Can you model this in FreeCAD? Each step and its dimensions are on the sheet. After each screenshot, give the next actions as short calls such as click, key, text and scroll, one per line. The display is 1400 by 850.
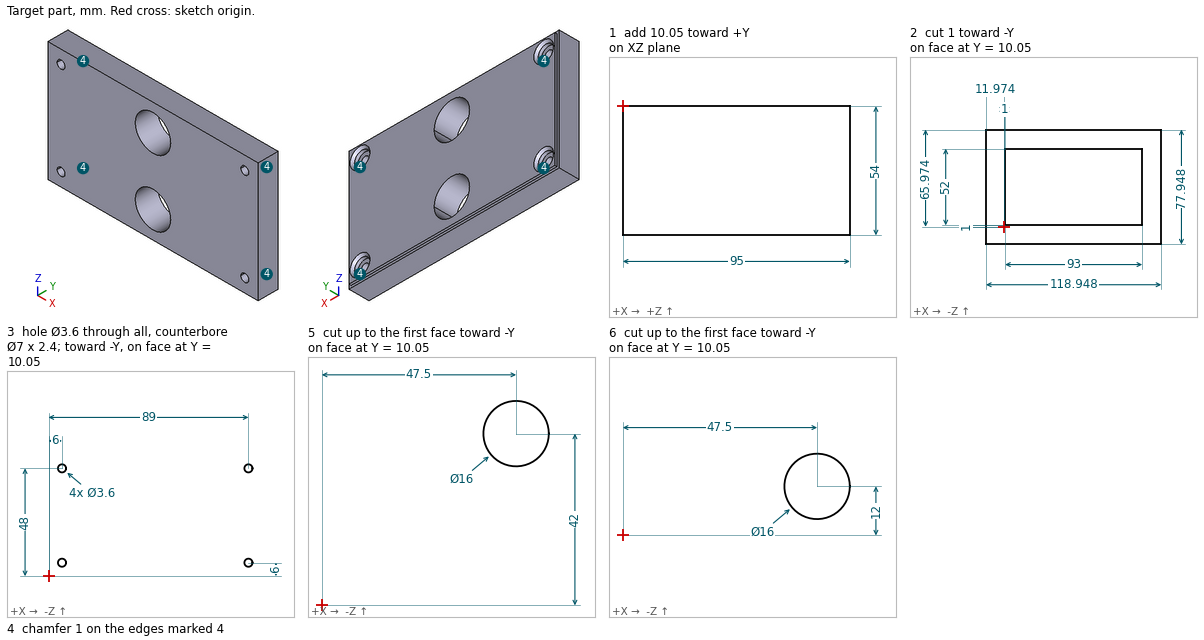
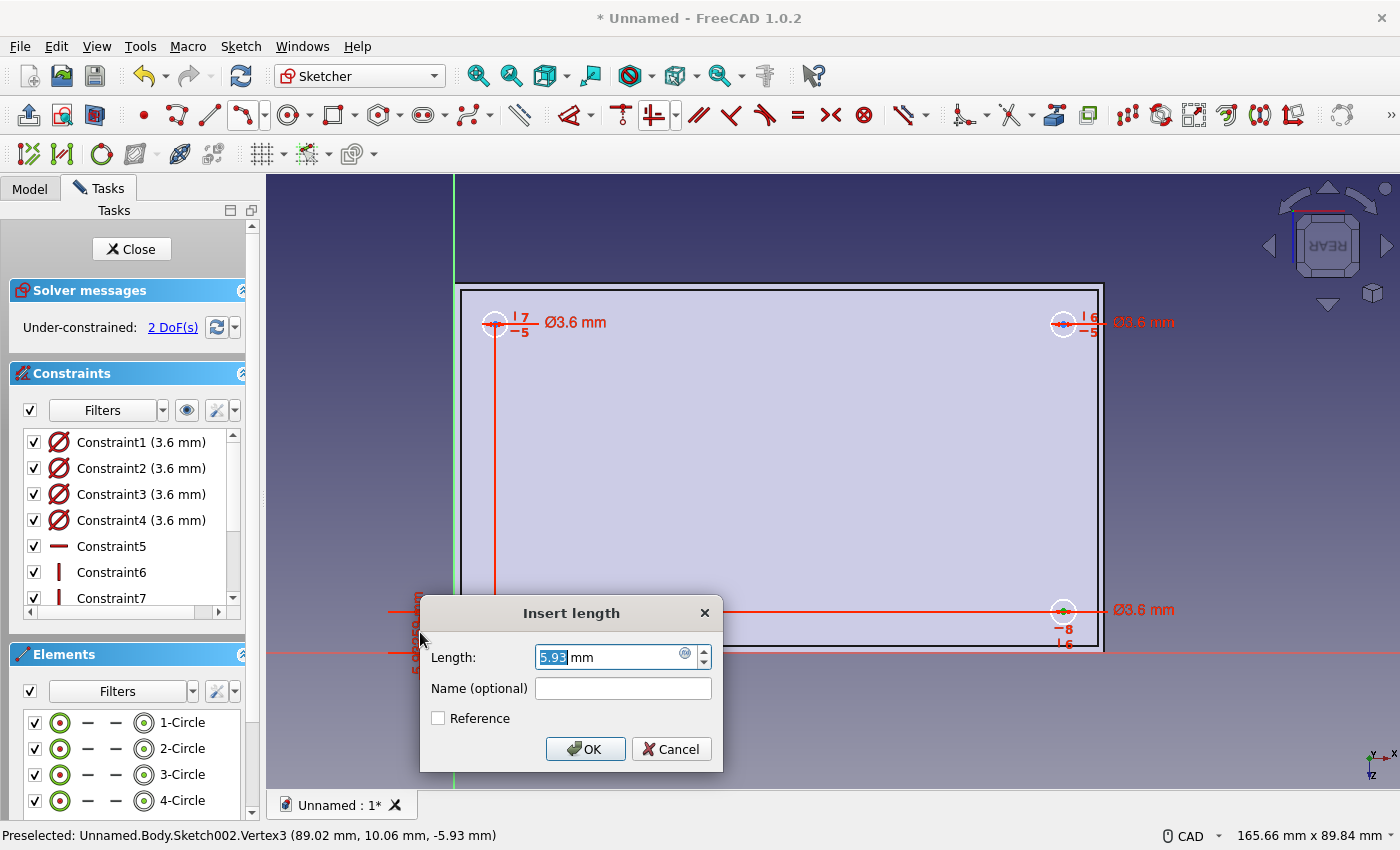
text(6)
key(Return)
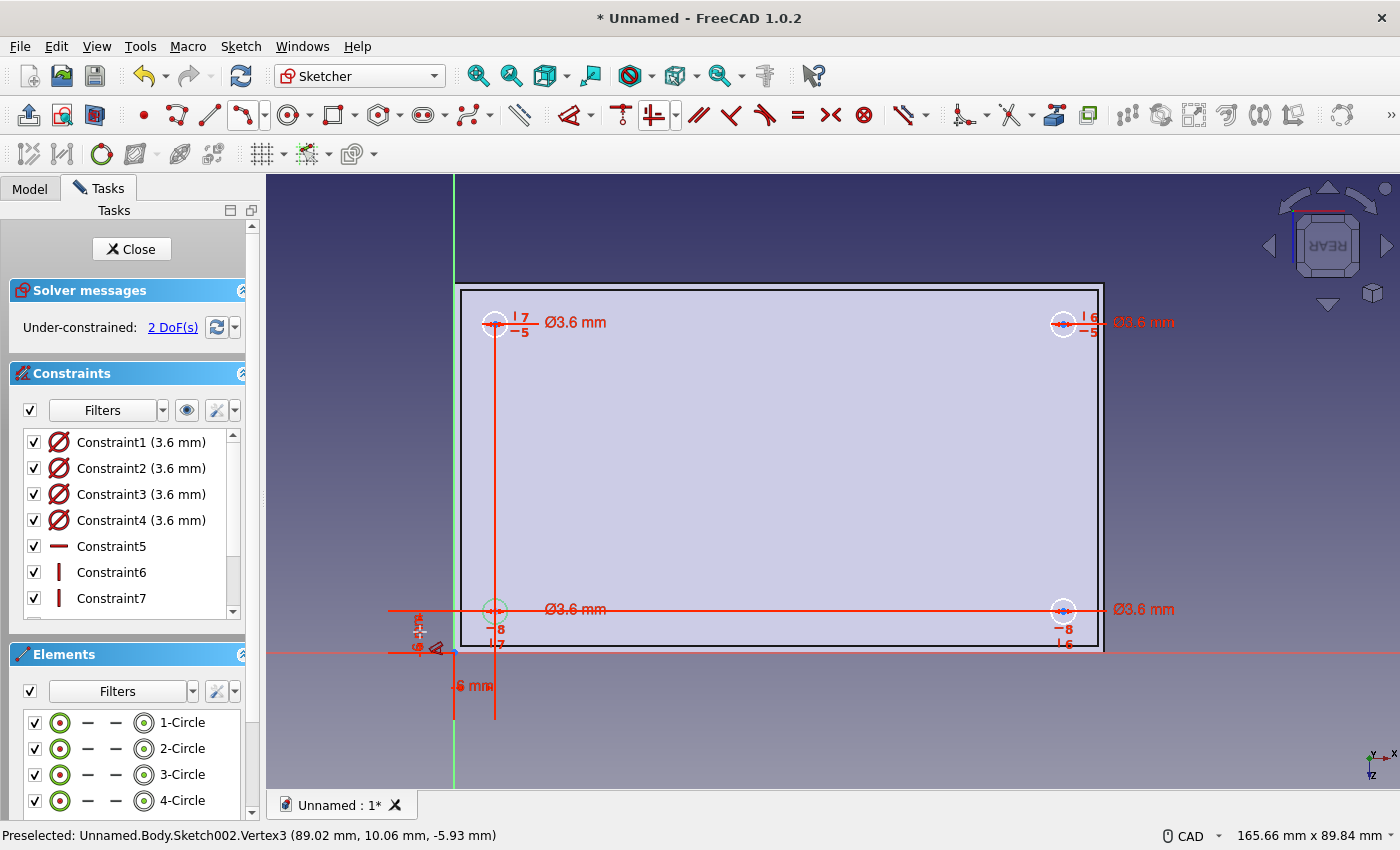
click(495, 324)
click(420, 489)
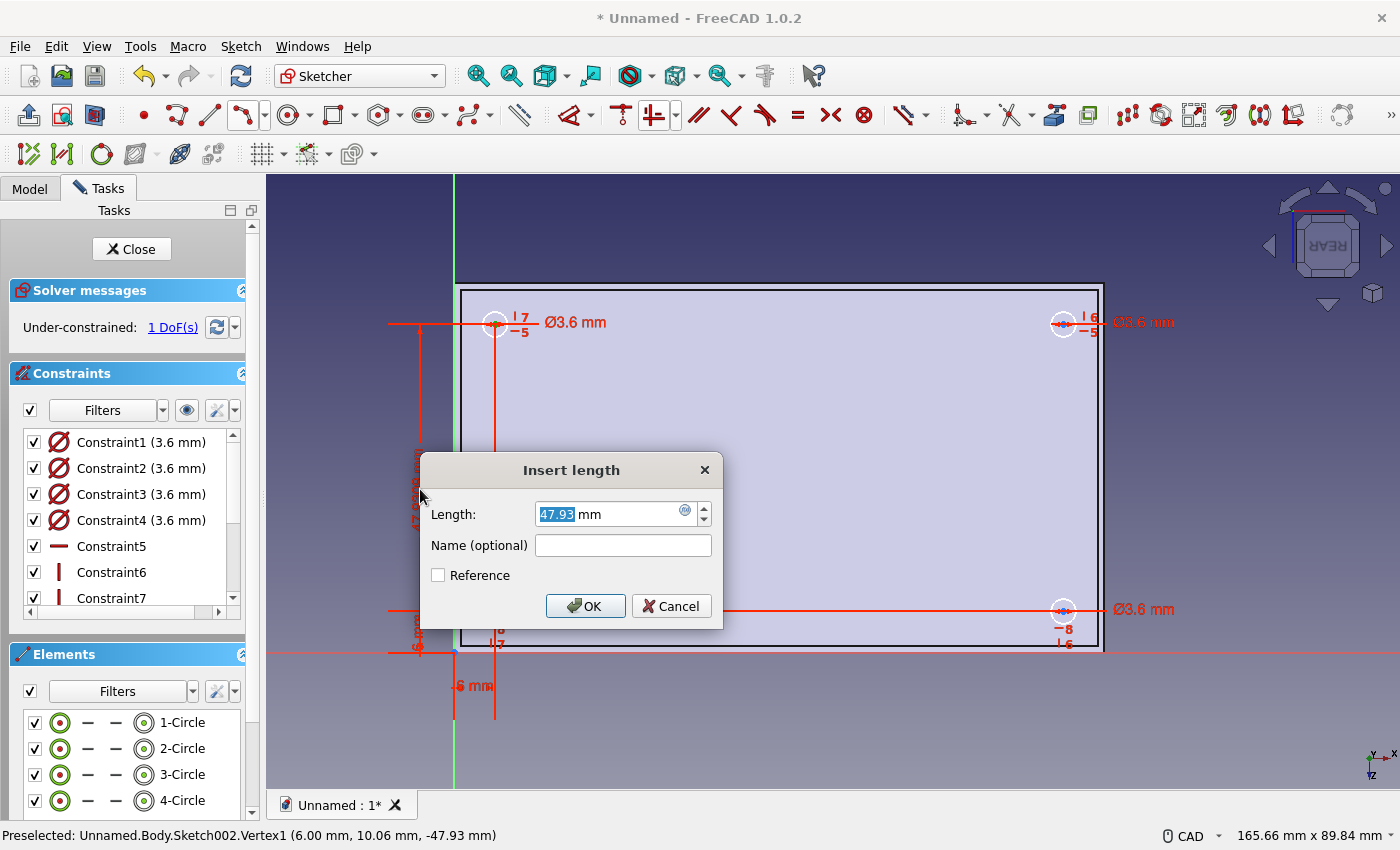
text(48)
key(Return)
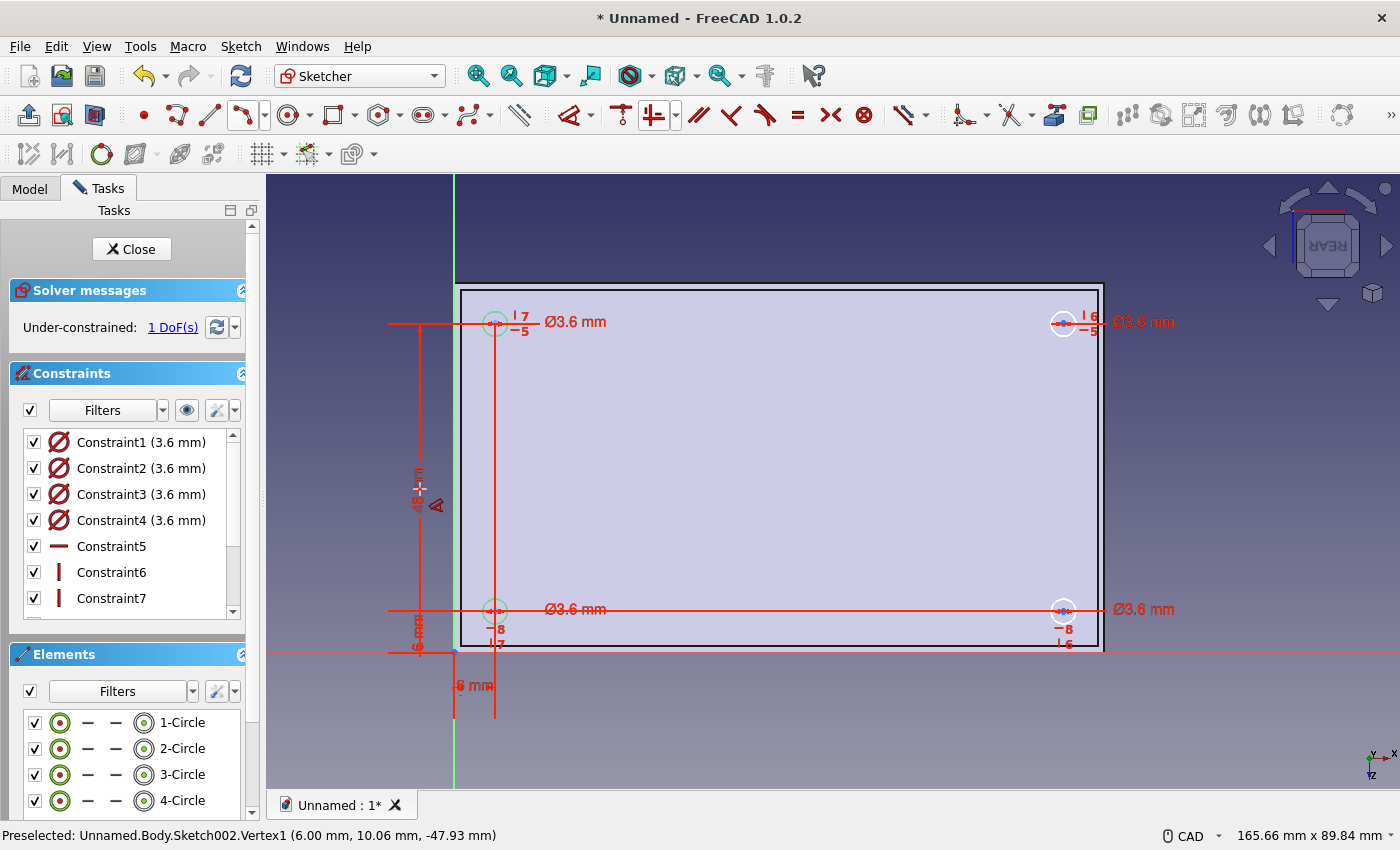
click(1063, 324)
click(759, 687)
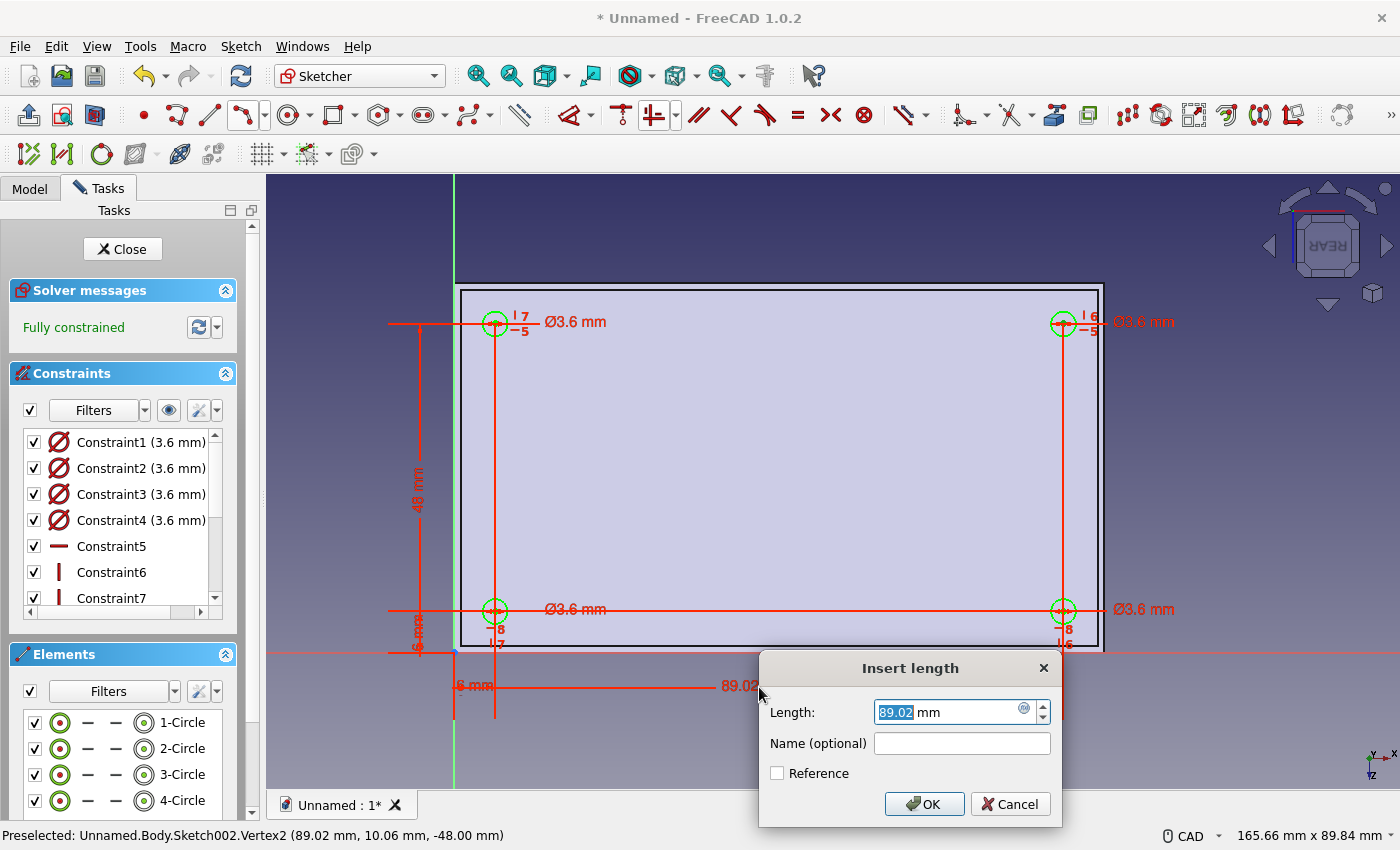
text(89)
key(Return)
key(Escape)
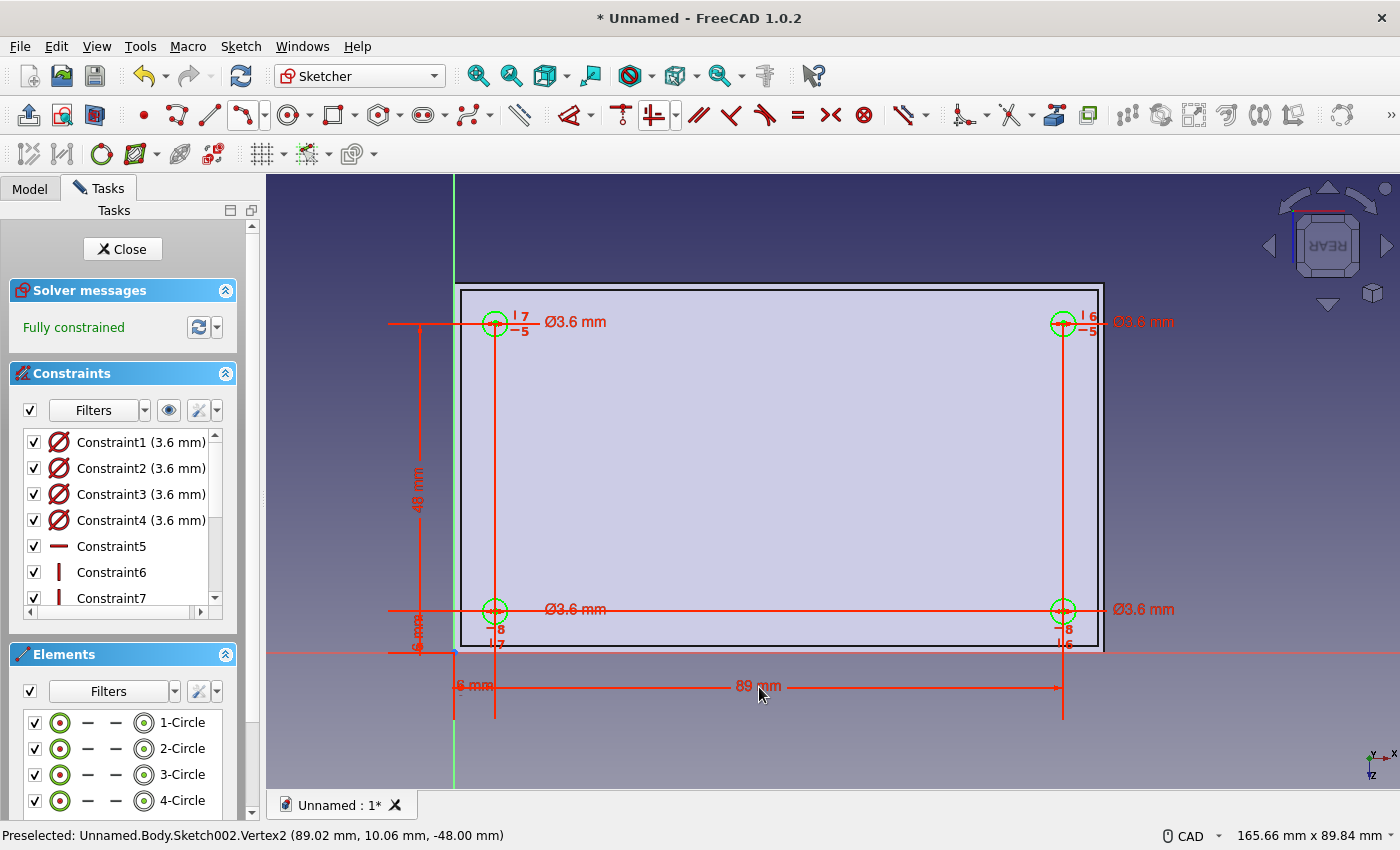
click(123, 249)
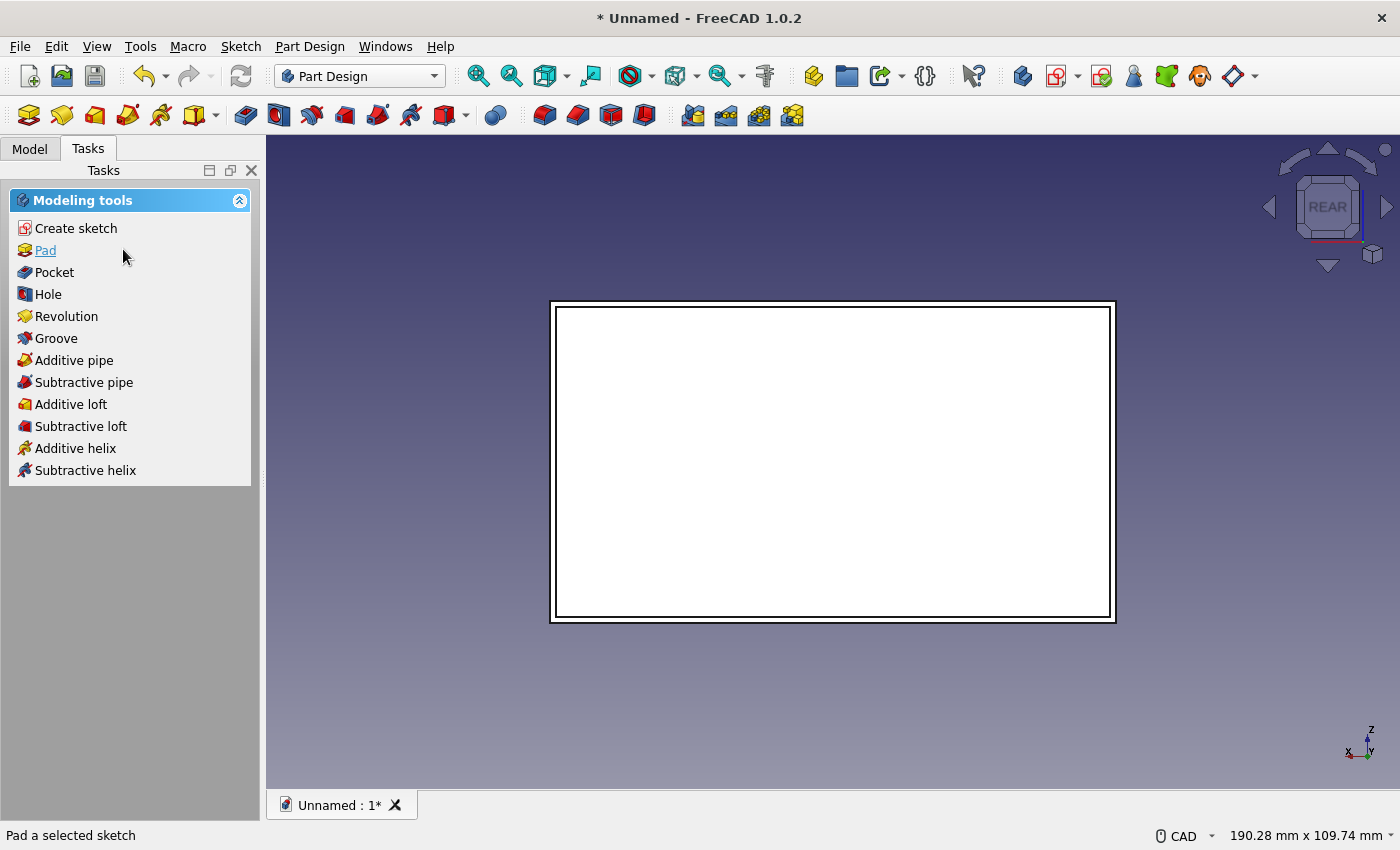
click(279, 116)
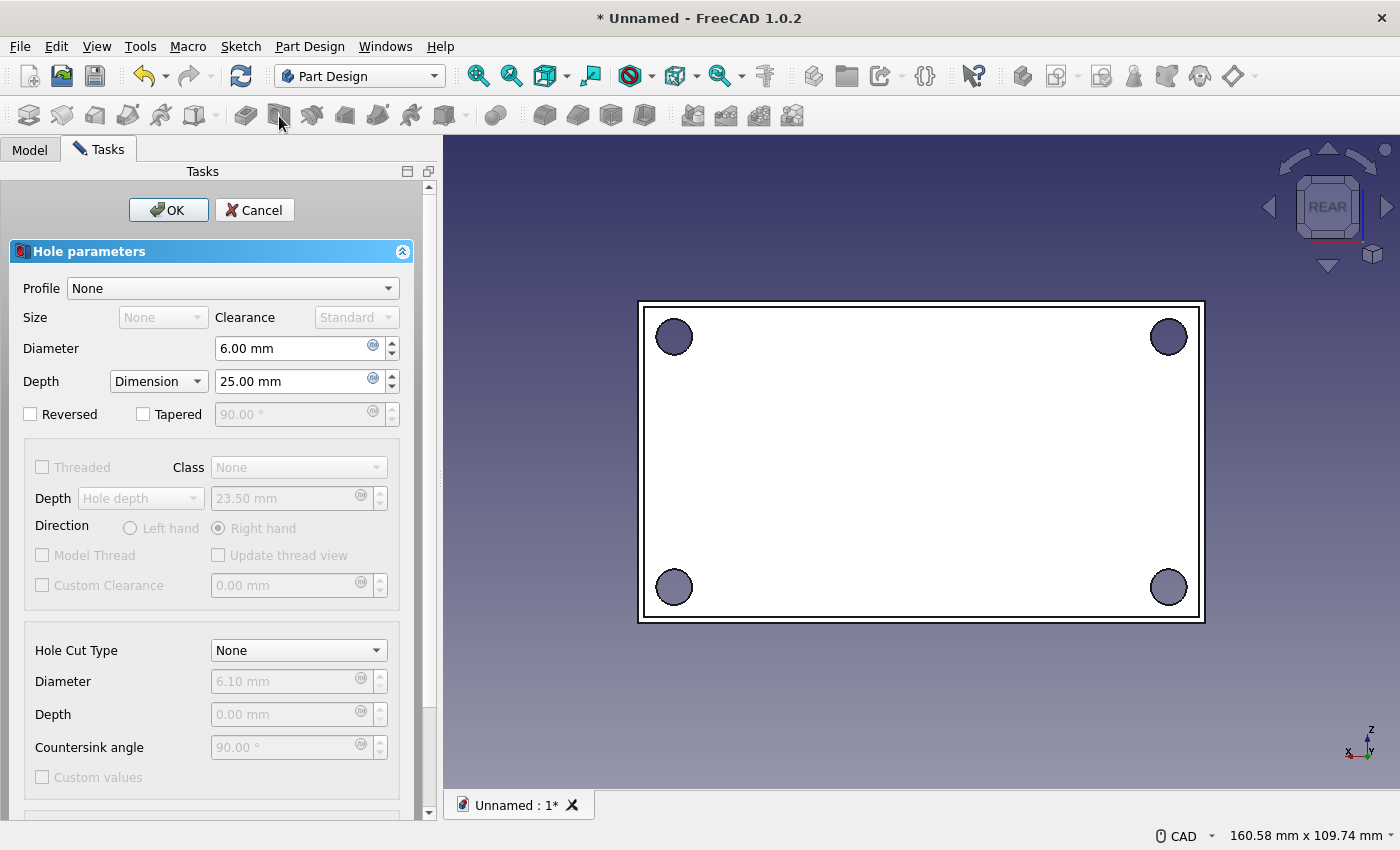
triple_click(300, 348)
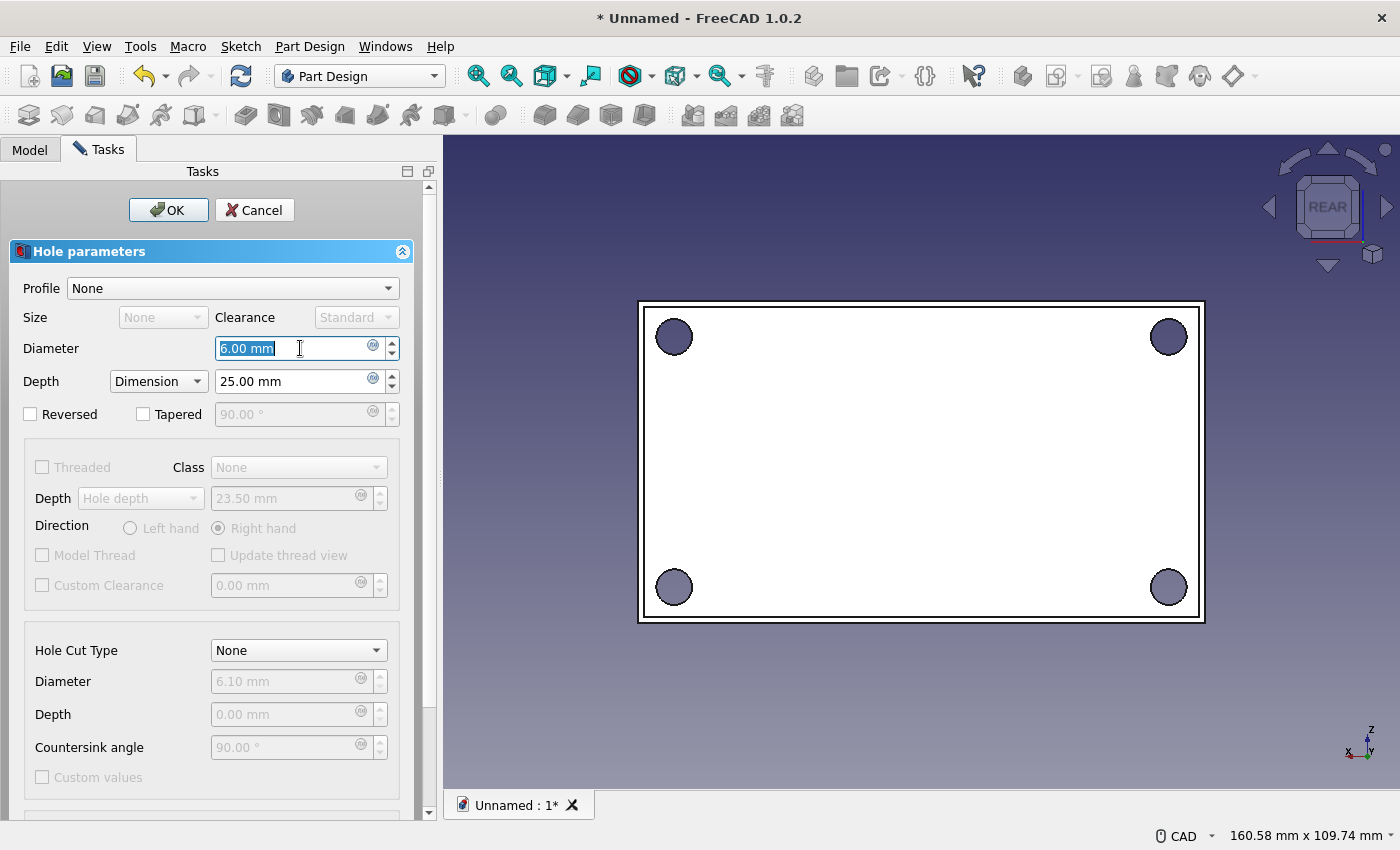
text(3.6)
key(Tab)